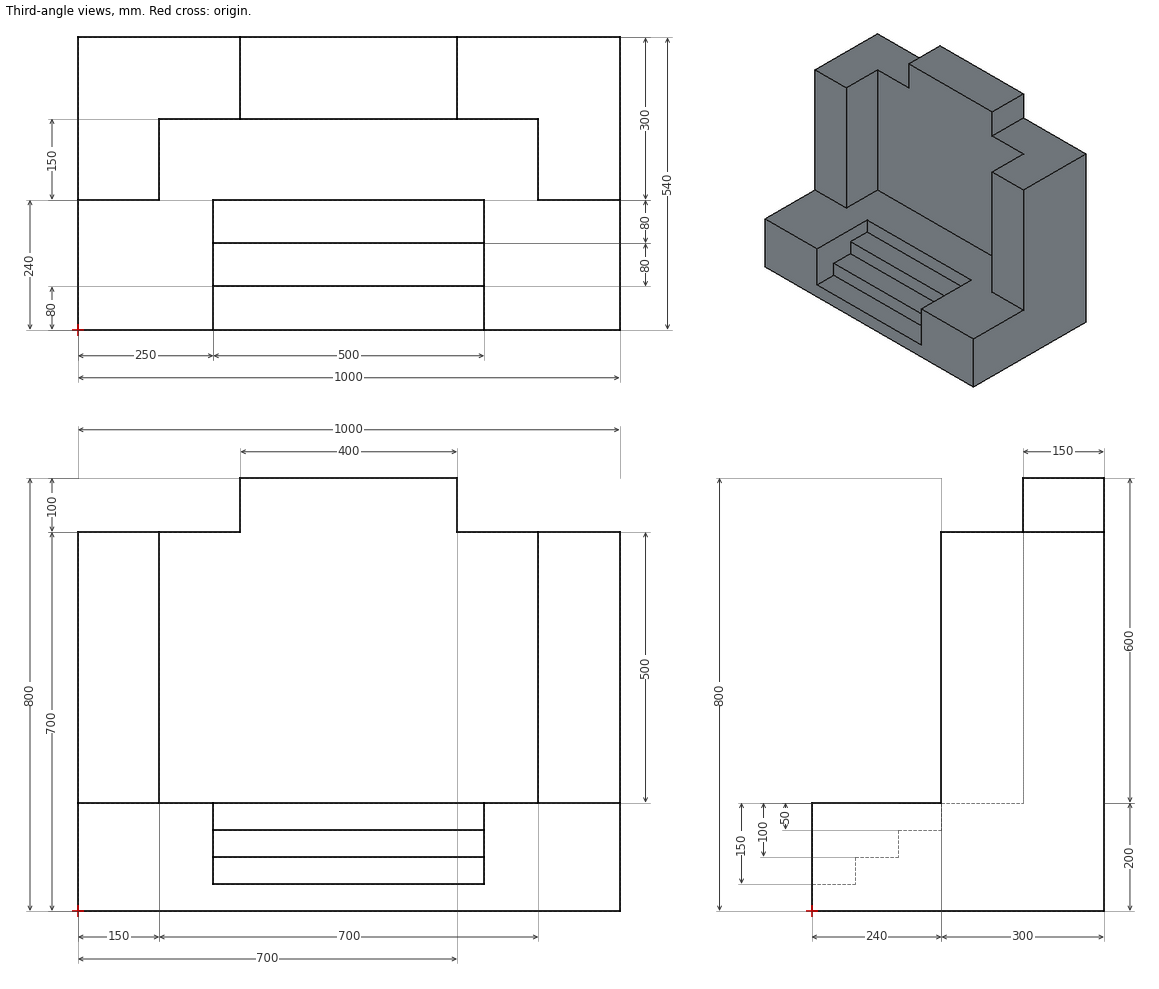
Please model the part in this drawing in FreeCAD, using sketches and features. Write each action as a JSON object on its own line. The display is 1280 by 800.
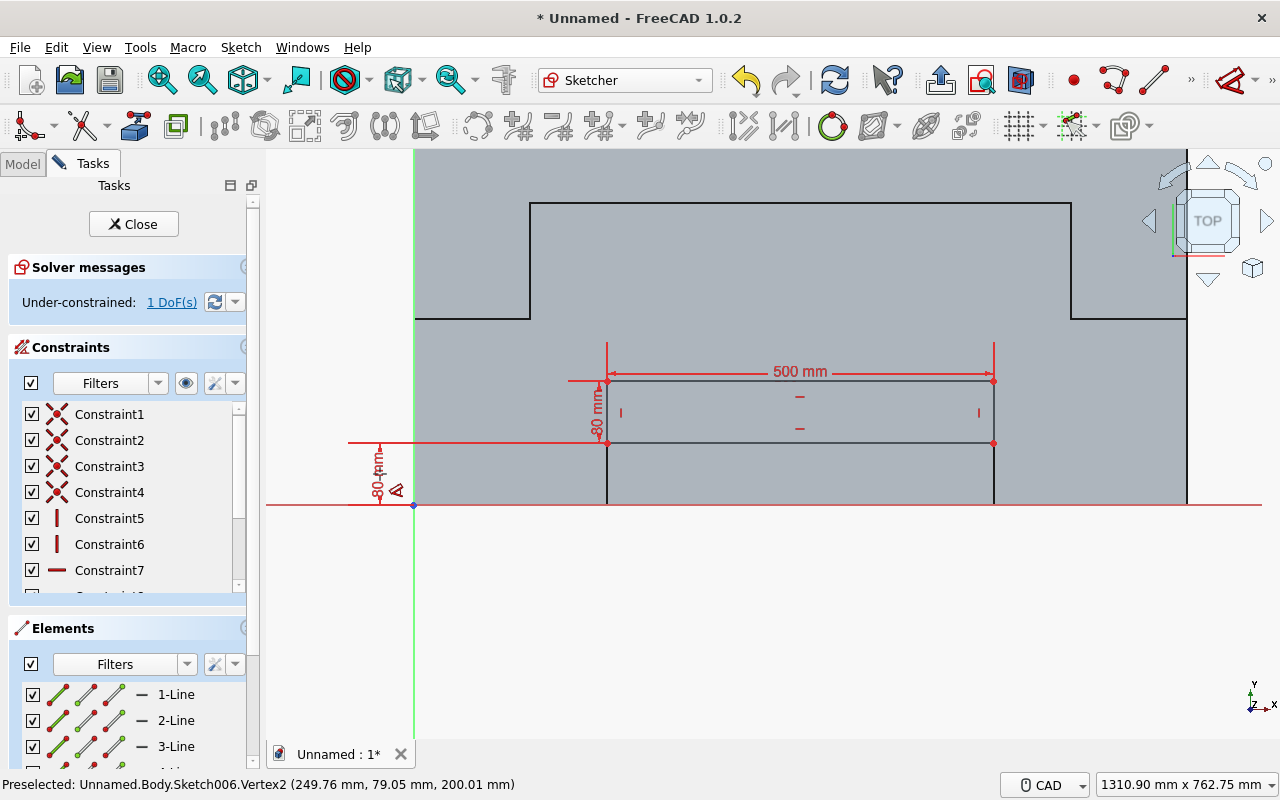
{"action": "left_click", "coordinate": [607, 381]}
{"action": "left_click", "coordinate": [510, 539]}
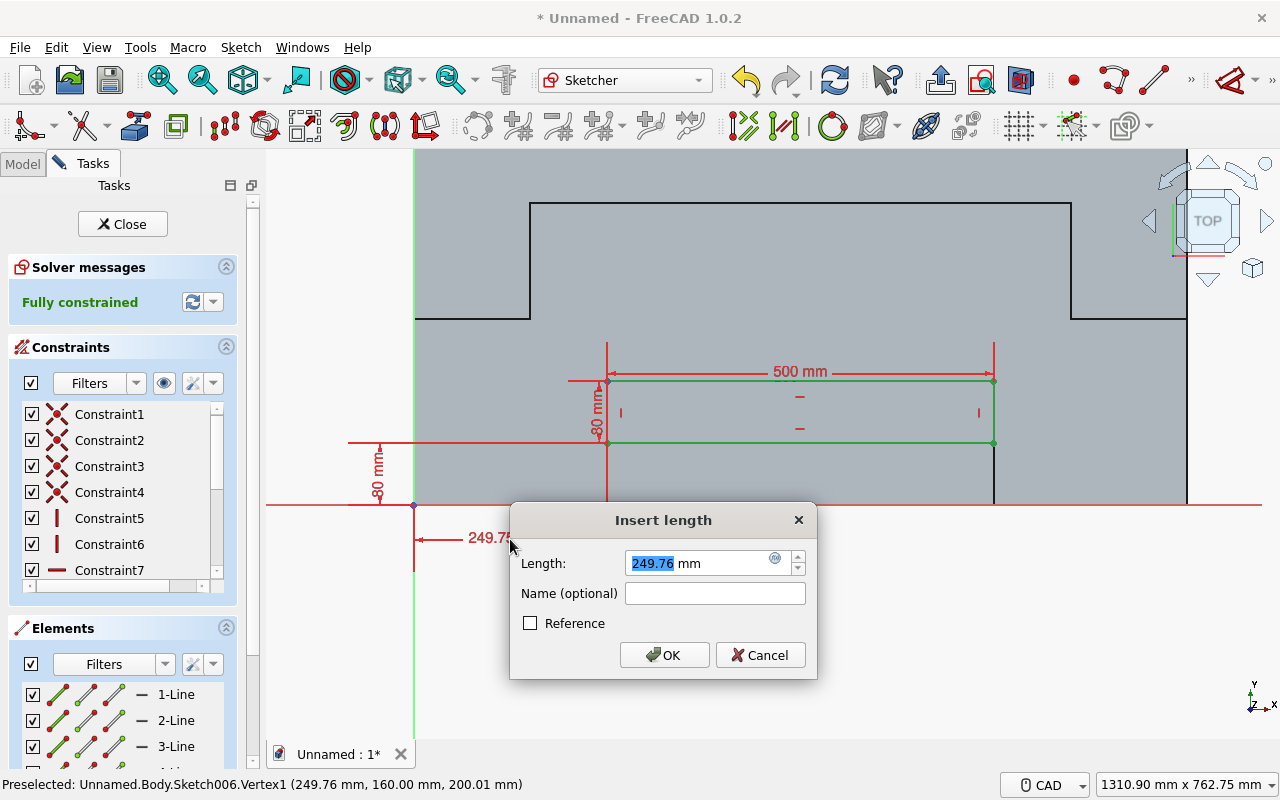
{"action": "type", "text": "250"}
{"action": "key", "text": "Return"}
{"action": "key", "text": "Escape"}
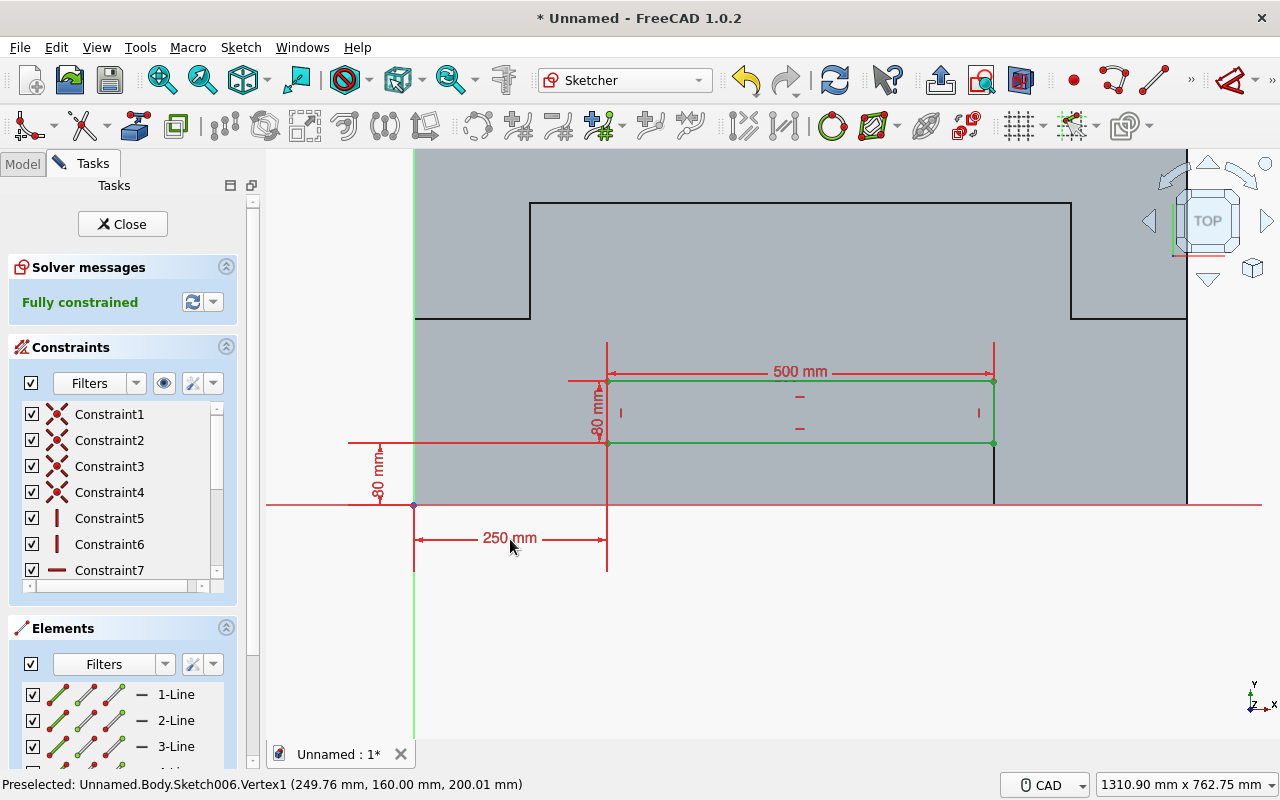
{"action": "left_click", "coordinate": [123, 224]}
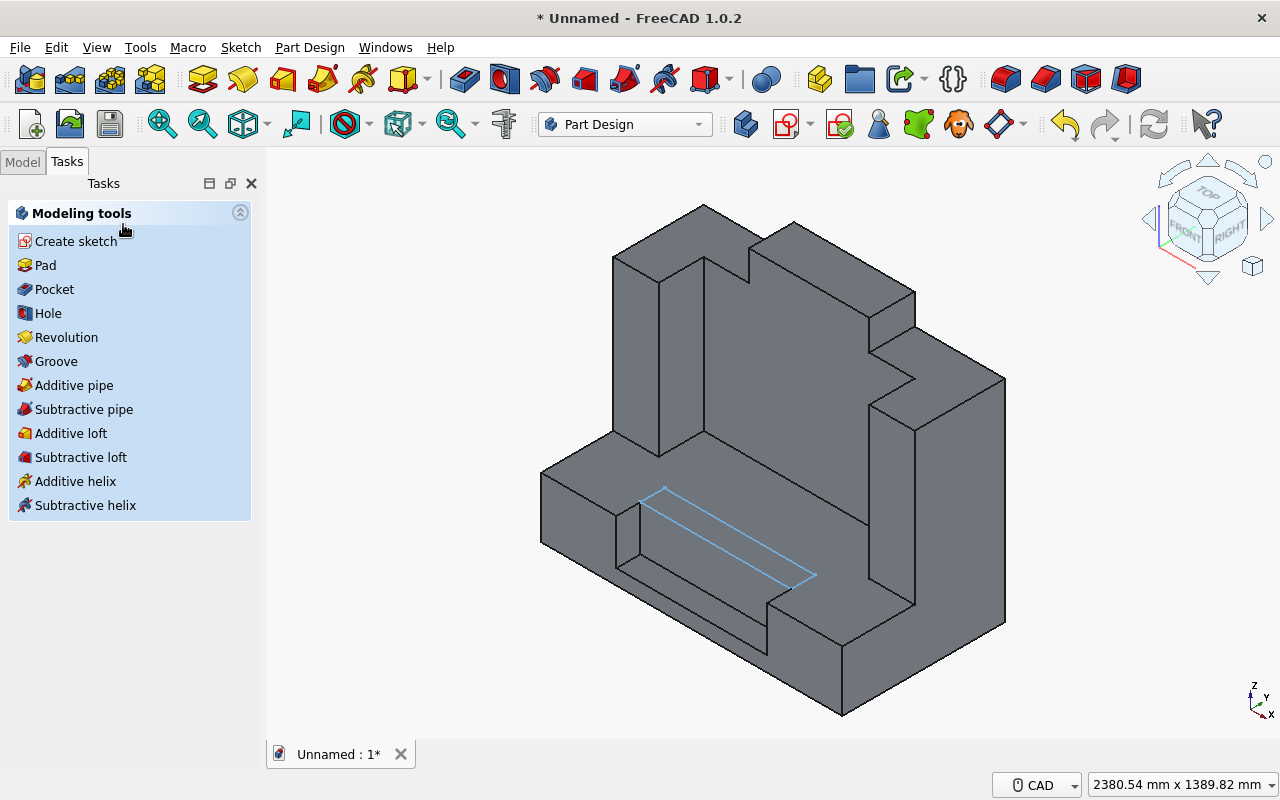
{"action": "left_click", "coordinate": [466, 80]}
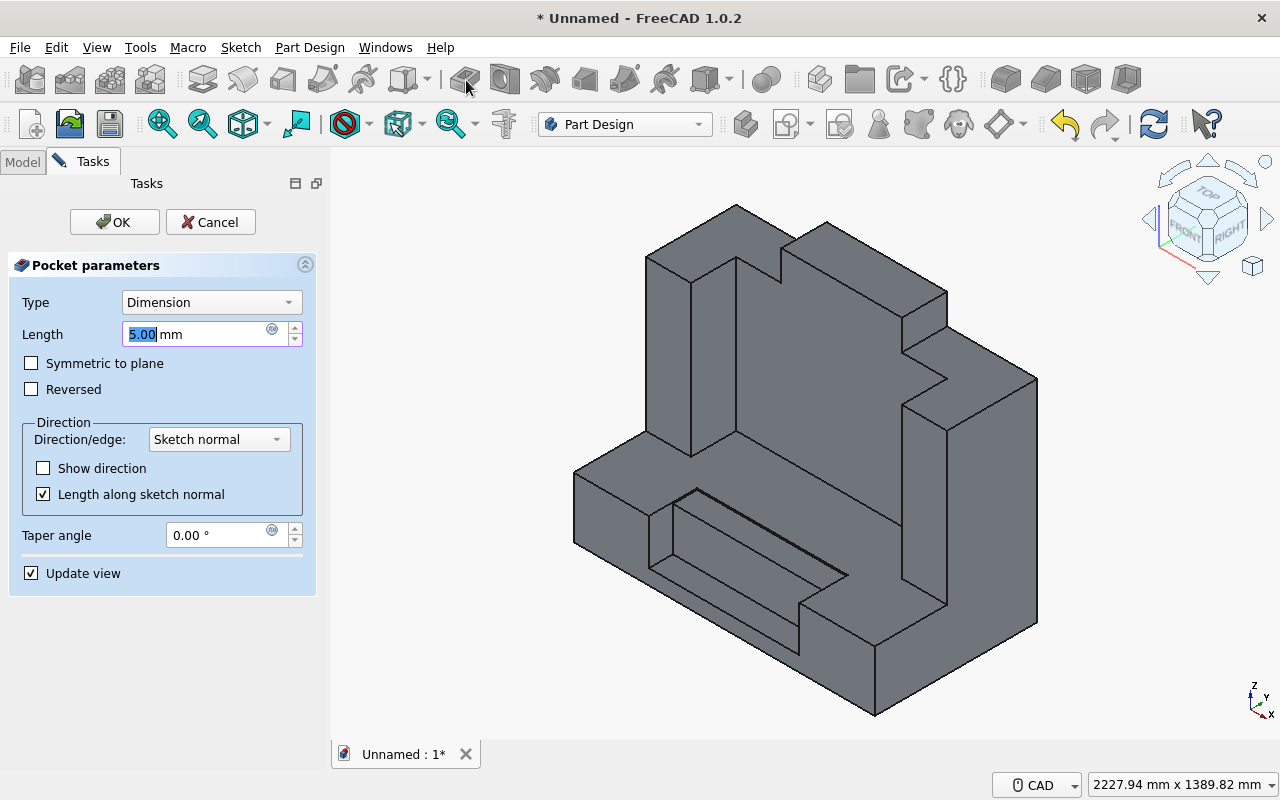
{"action": "type", "text": "100"}
{"action": "key", "text": "Tab"}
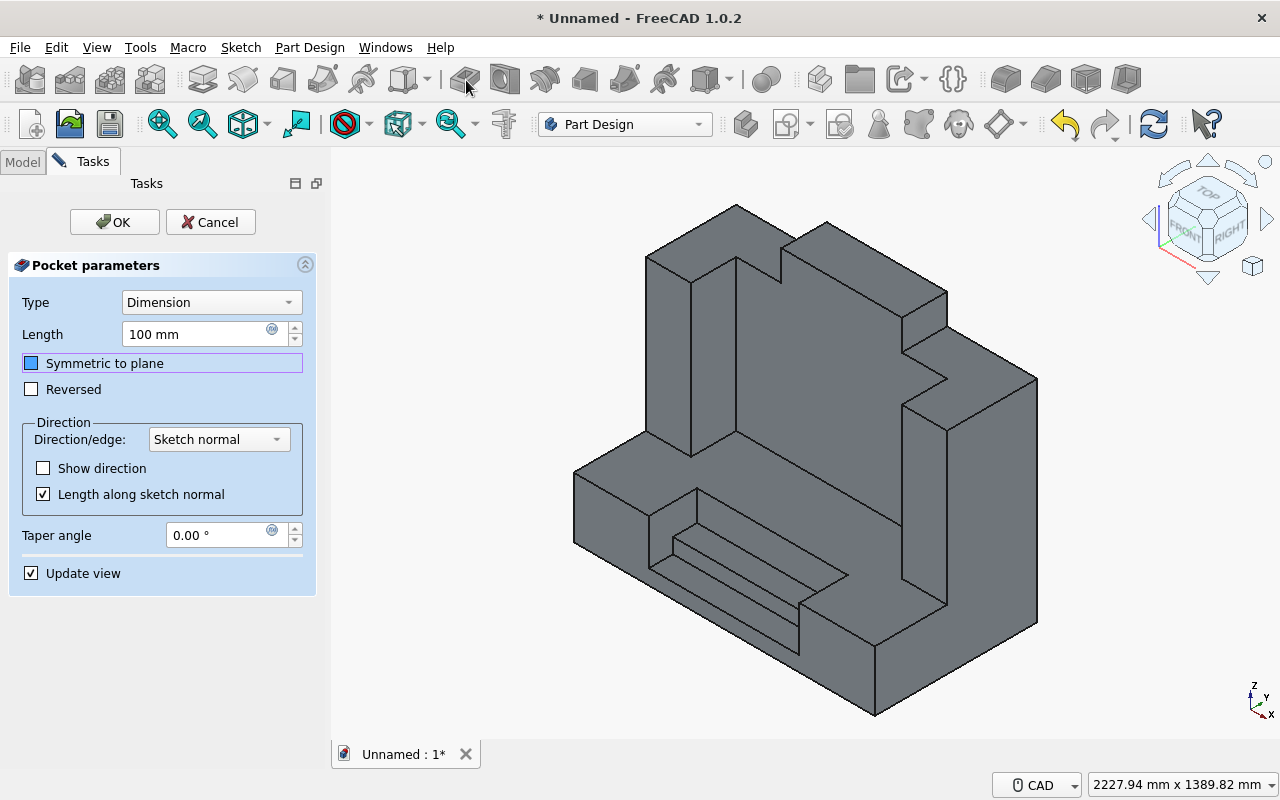
{"action": "left_click", "coordinate": [115, 222]}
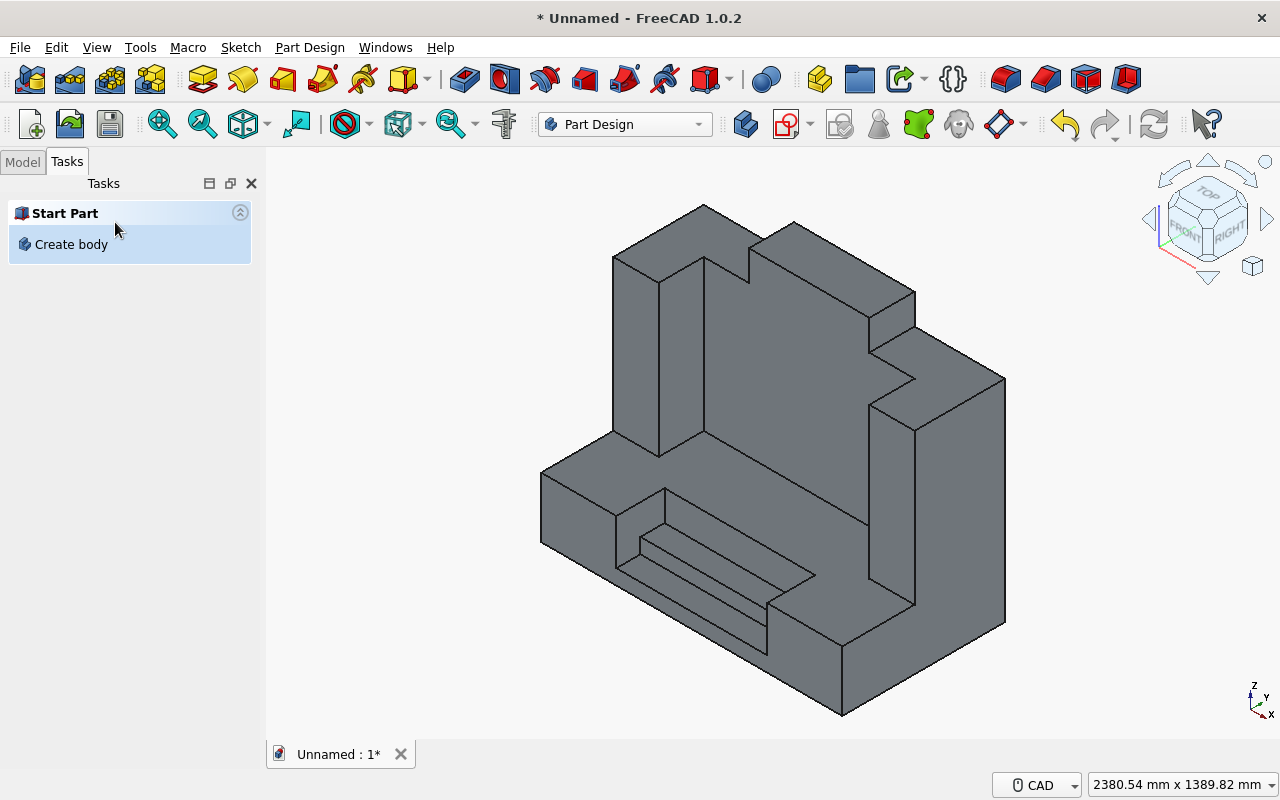
{"action": "left_click", "coordinate": [810, 540]}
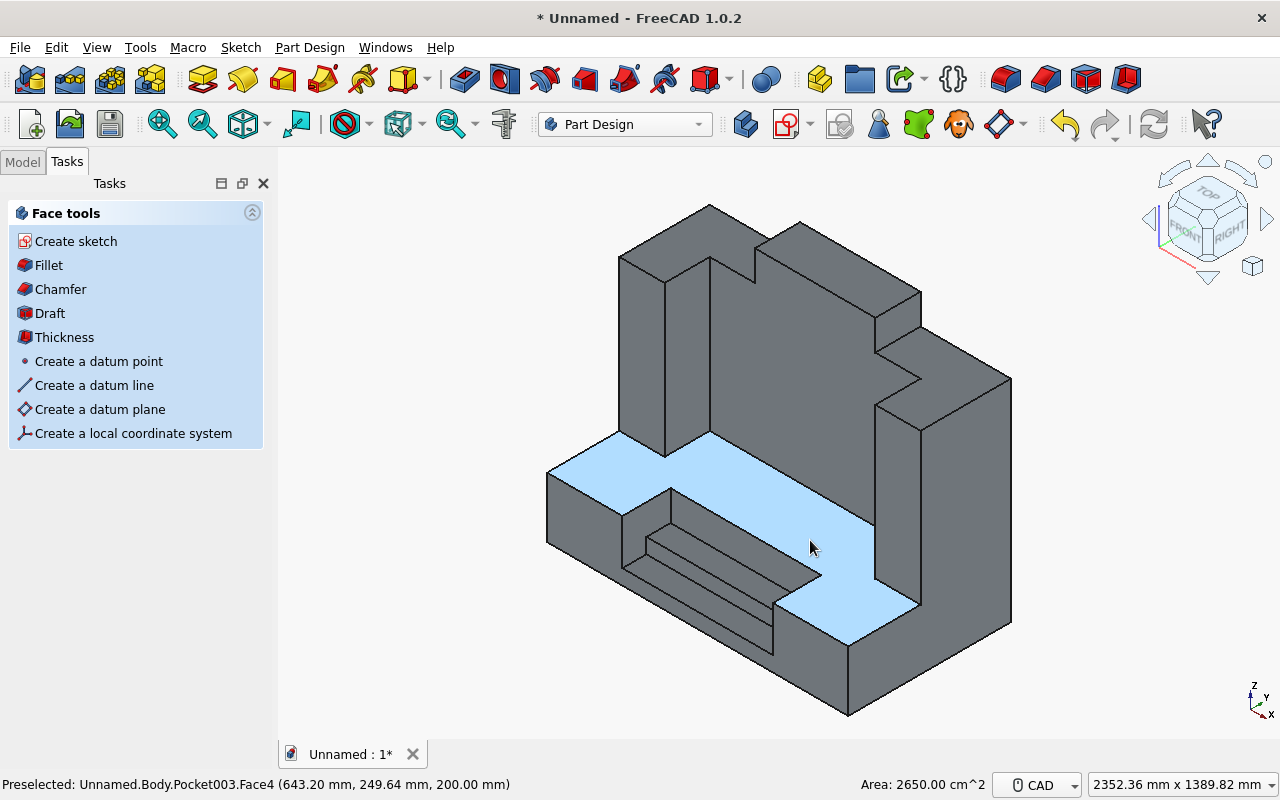
{"action": "left_click", "coordinate": [786, 124]}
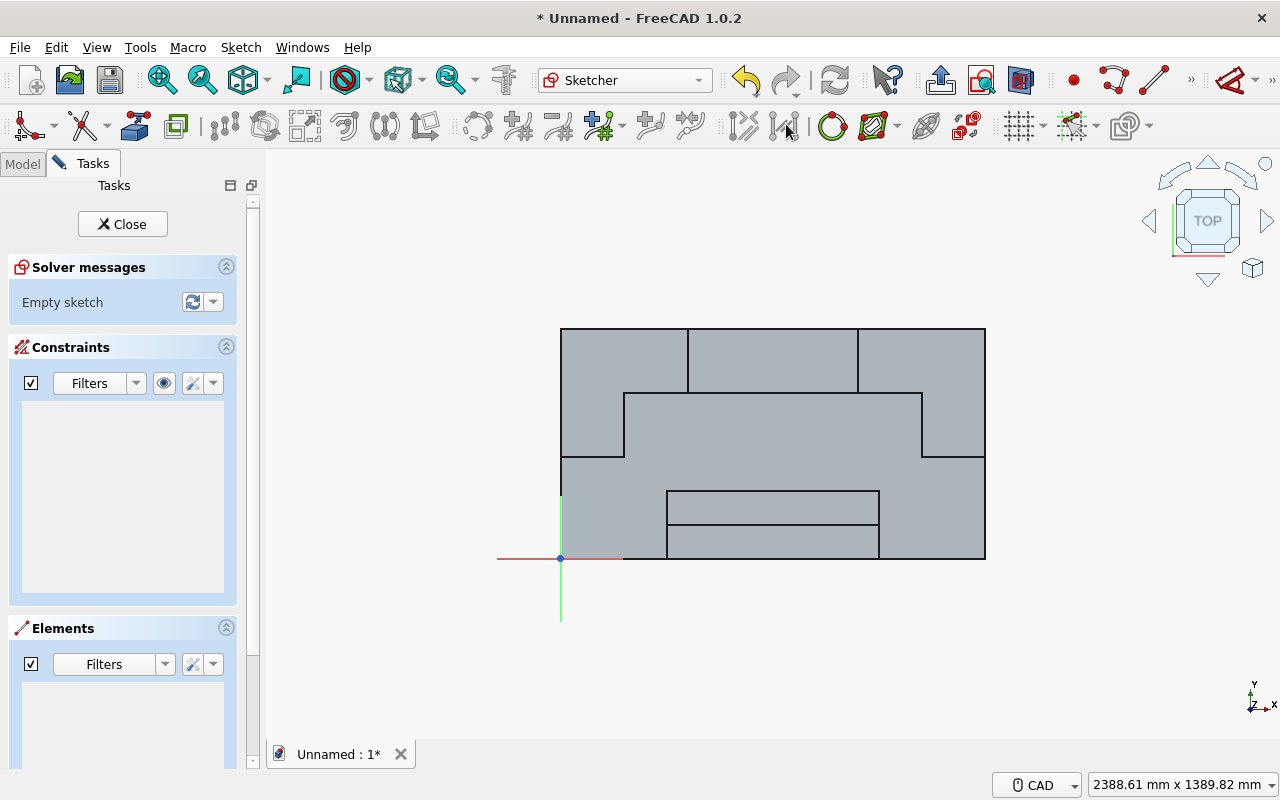
{"action": "left_click", "coordinate": [1022, 80]}